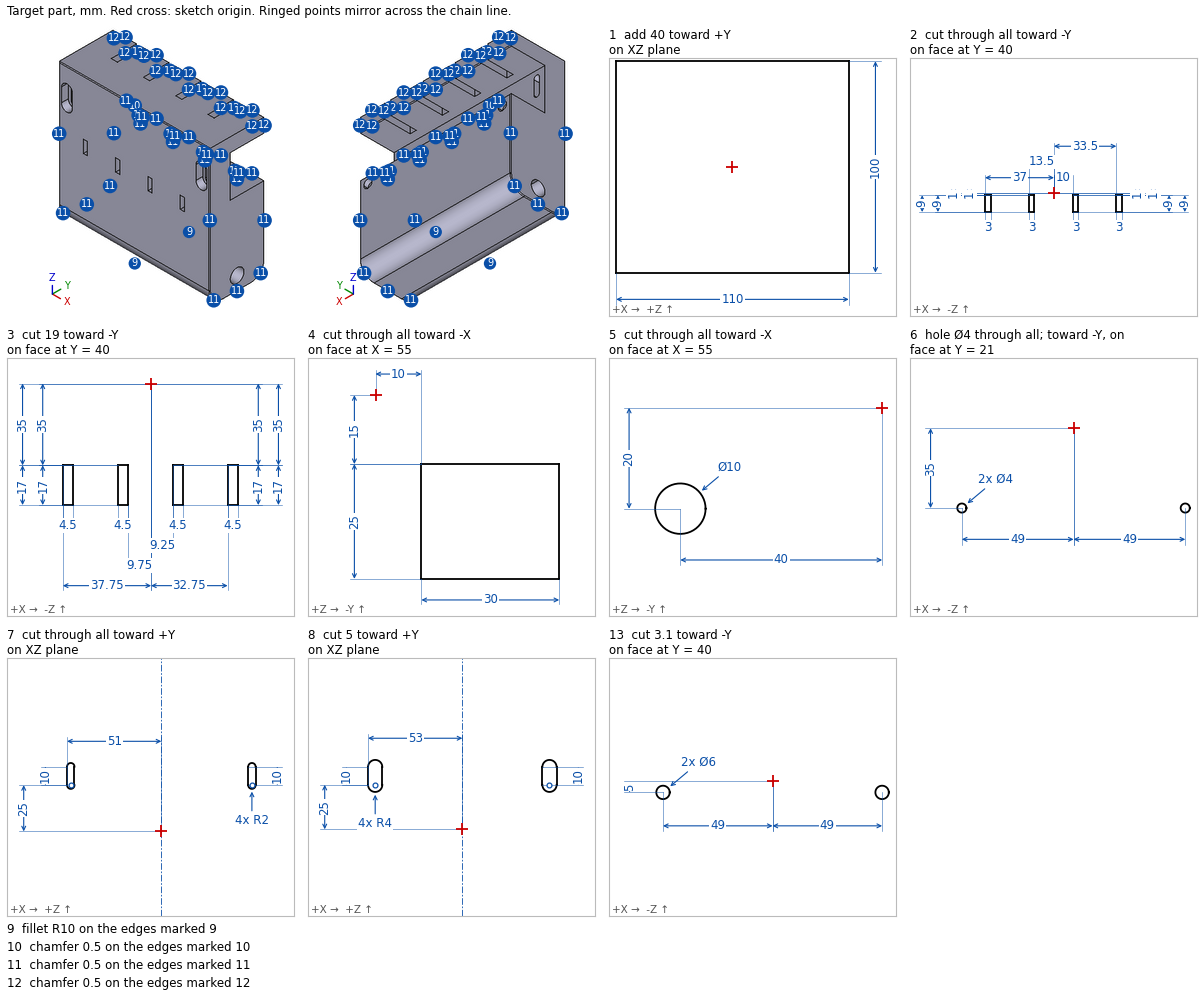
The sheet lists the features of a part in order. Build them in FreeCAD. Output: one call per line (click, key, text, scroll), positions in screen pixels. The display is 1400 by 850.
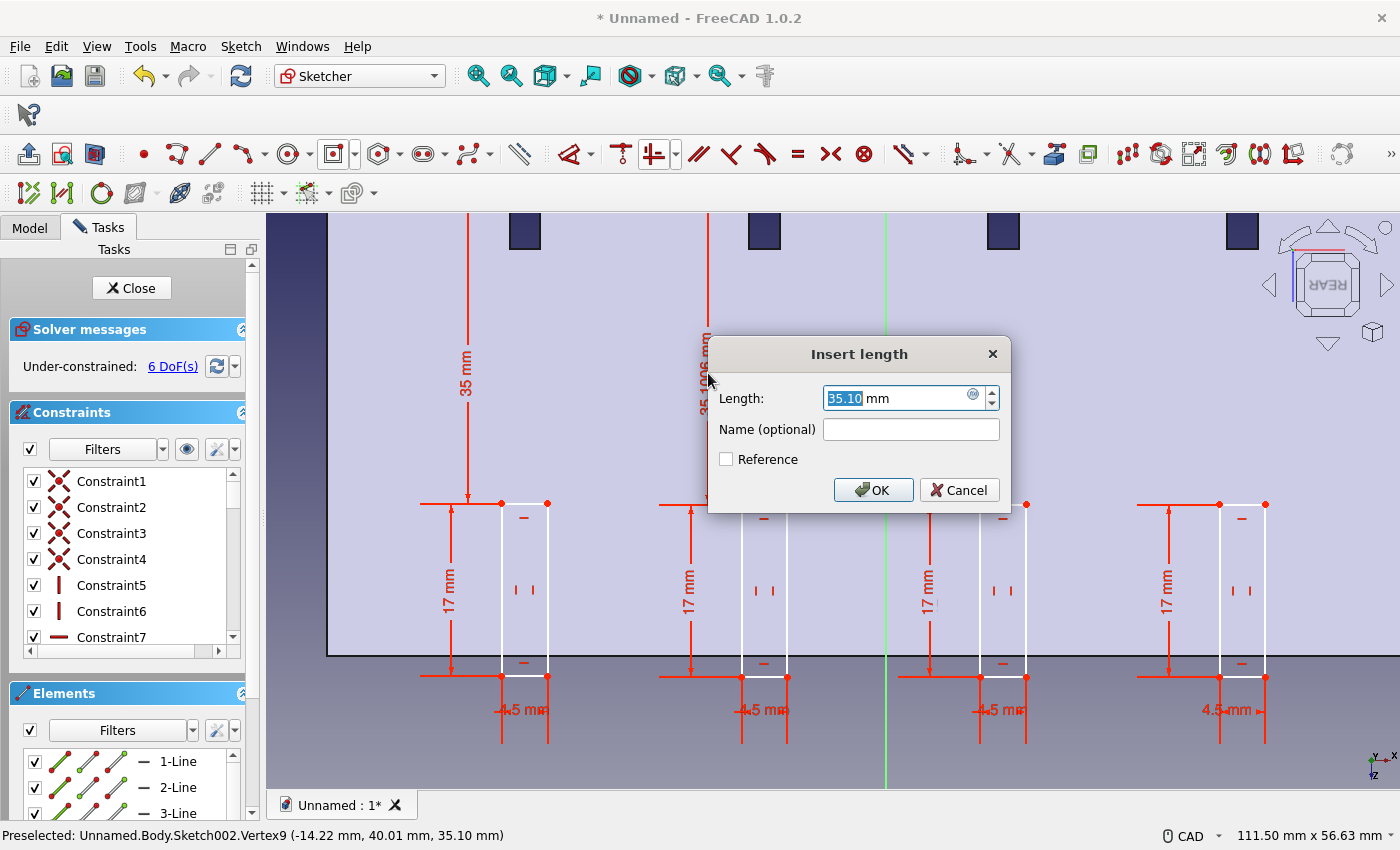
text(35)
key(Return)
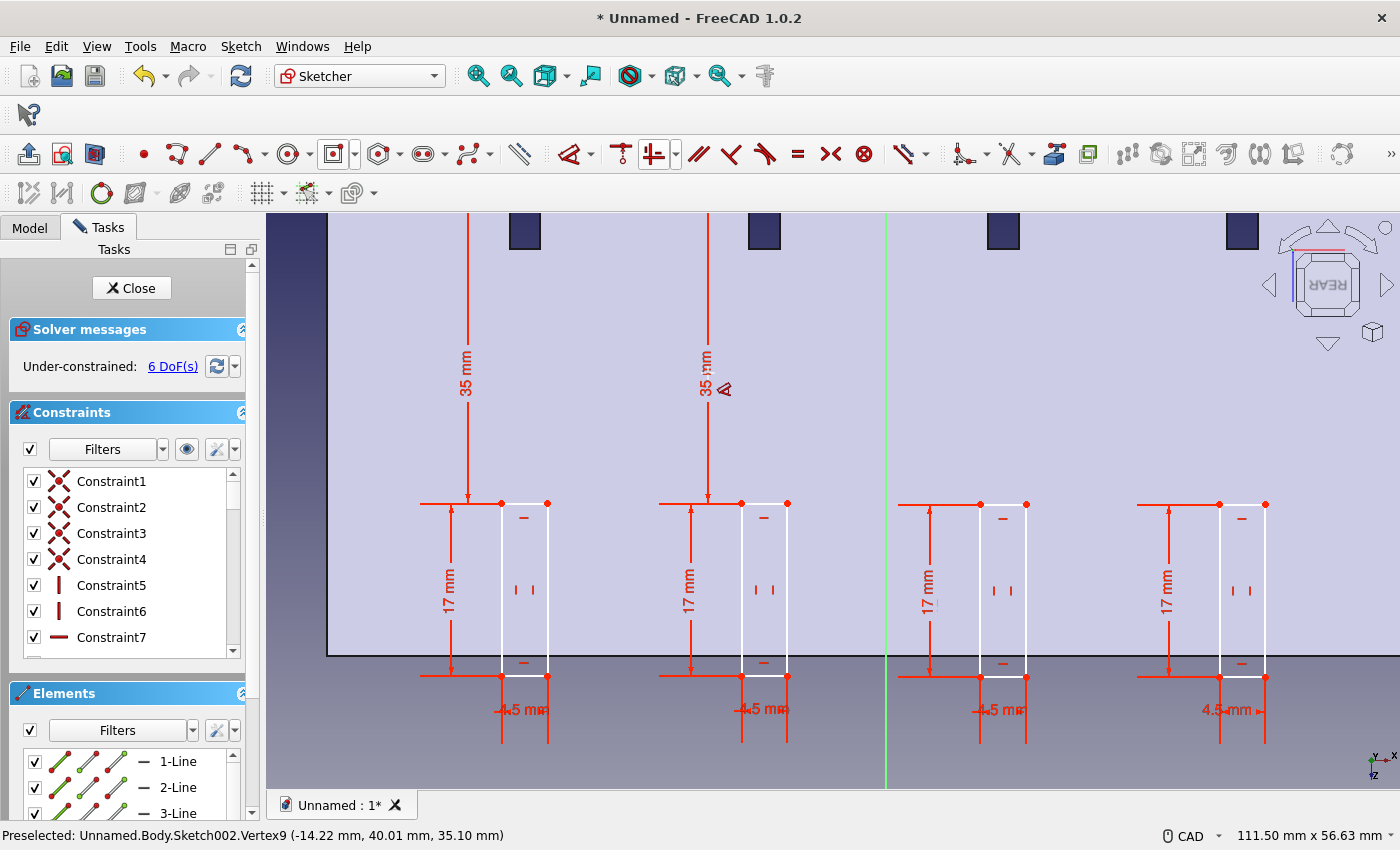
click(980, 505)
click(1014, 373)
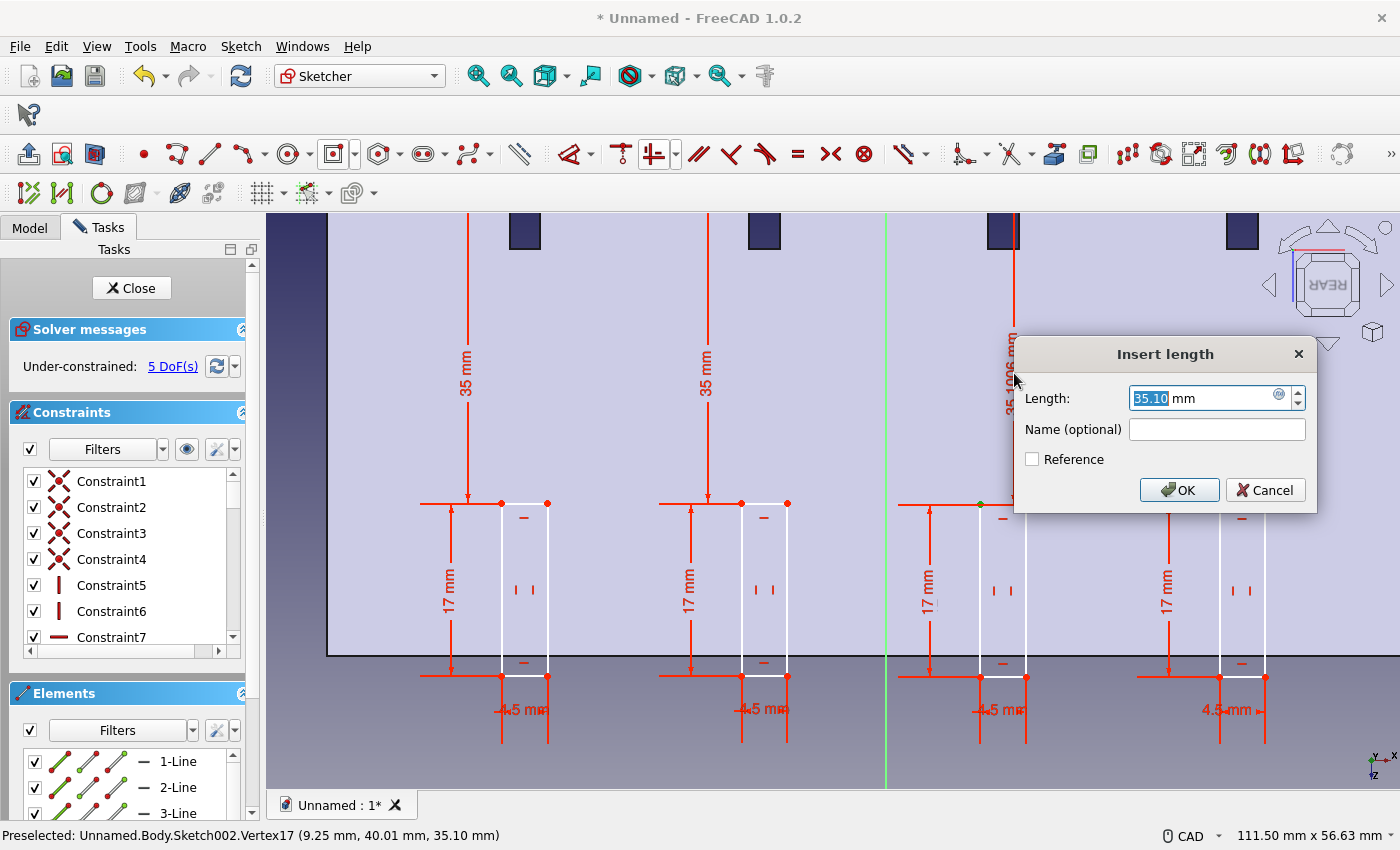
text(35)
key(Return)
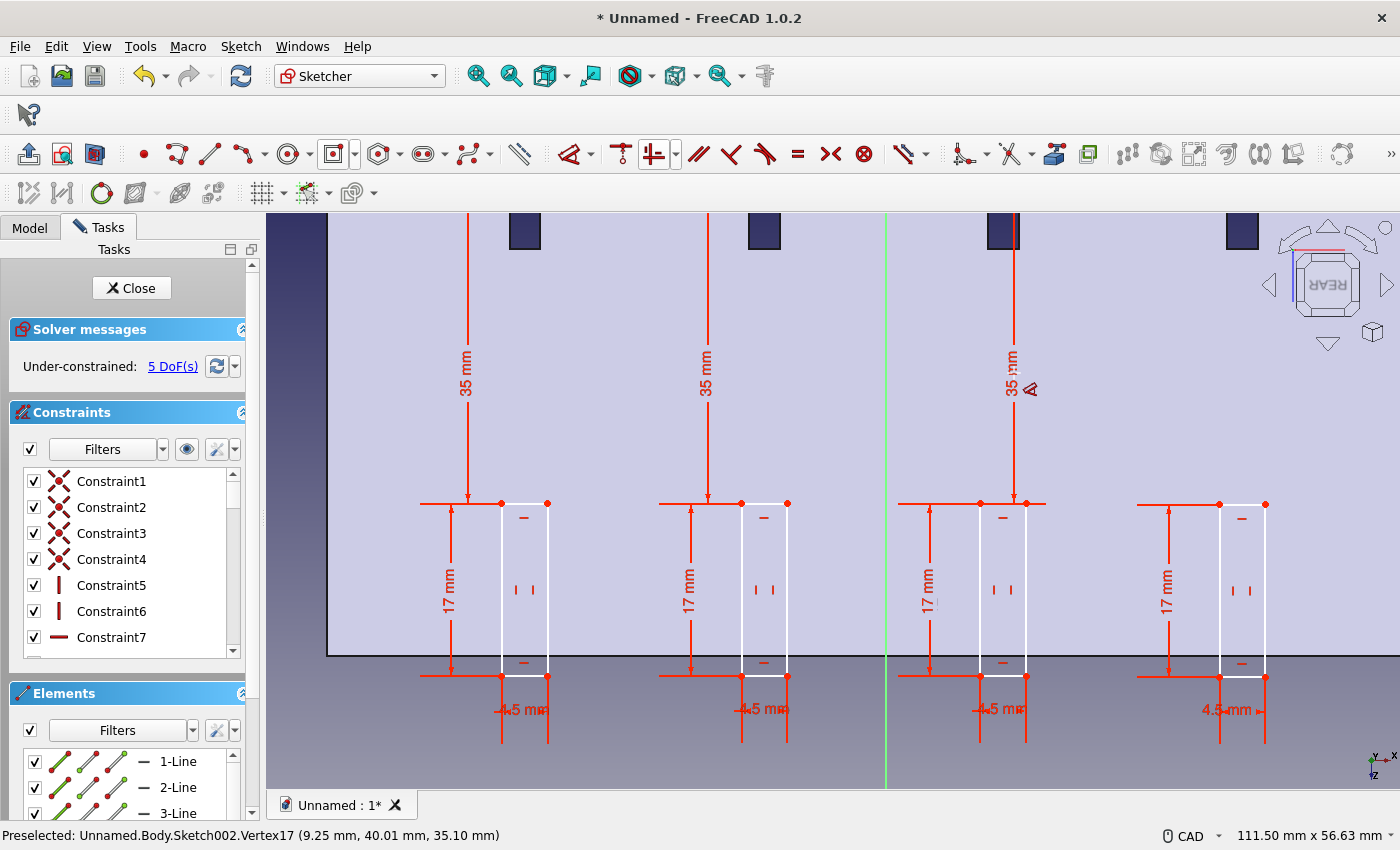
click(1220, 505)
click(852, 373)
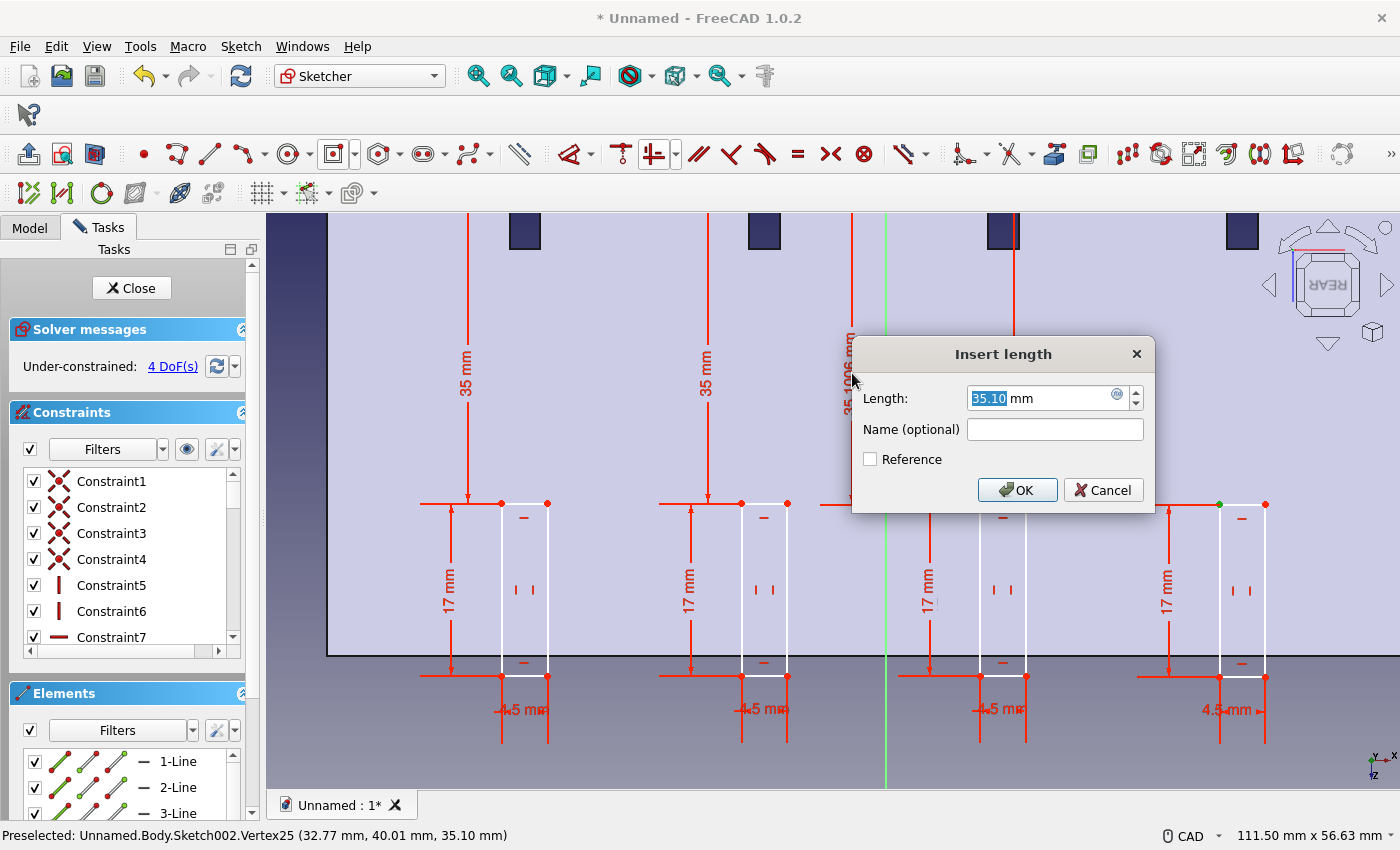
text(35)
key(Return)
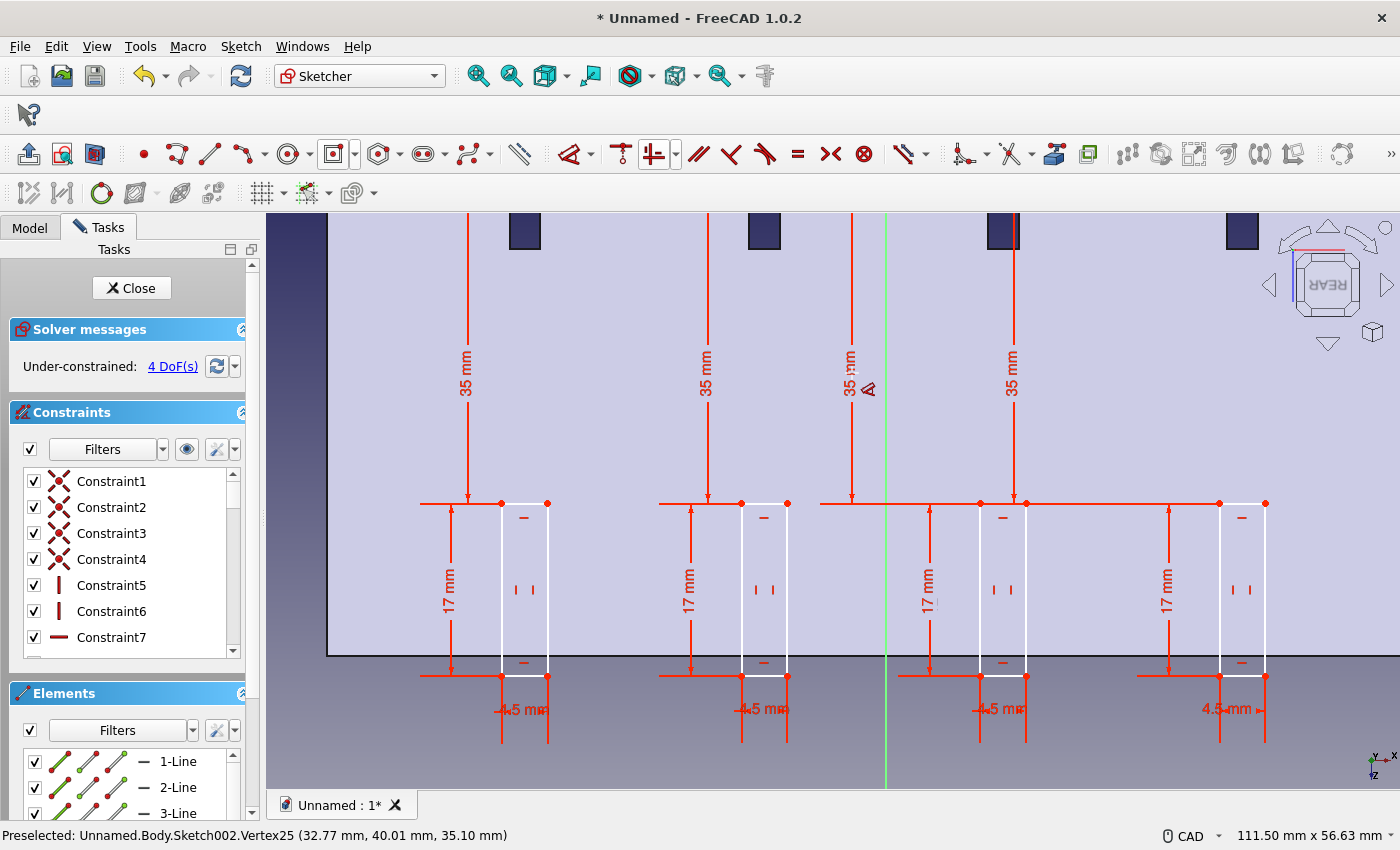
click(787, 676)
click(837, 710)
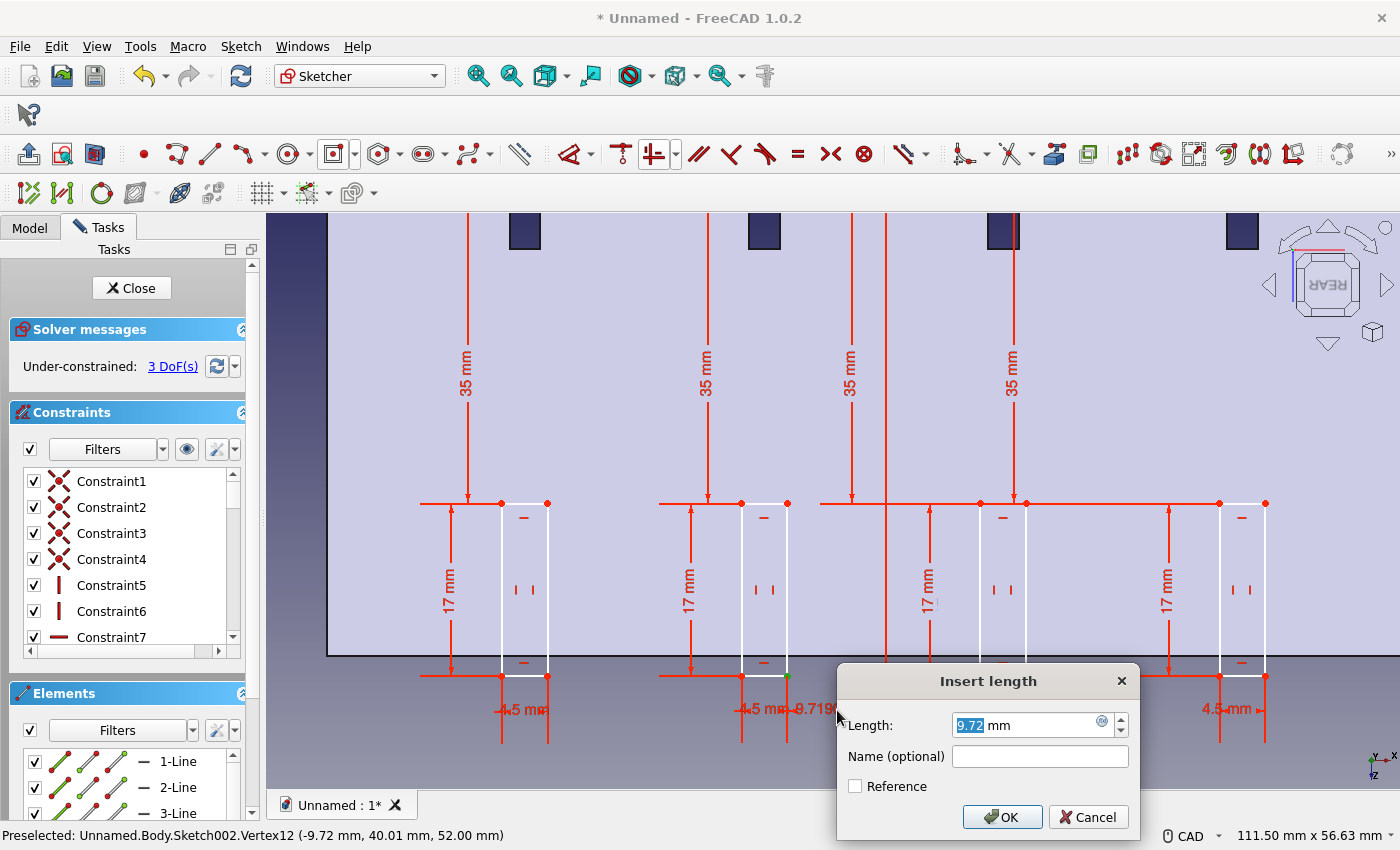
text(9.75)
key(Return)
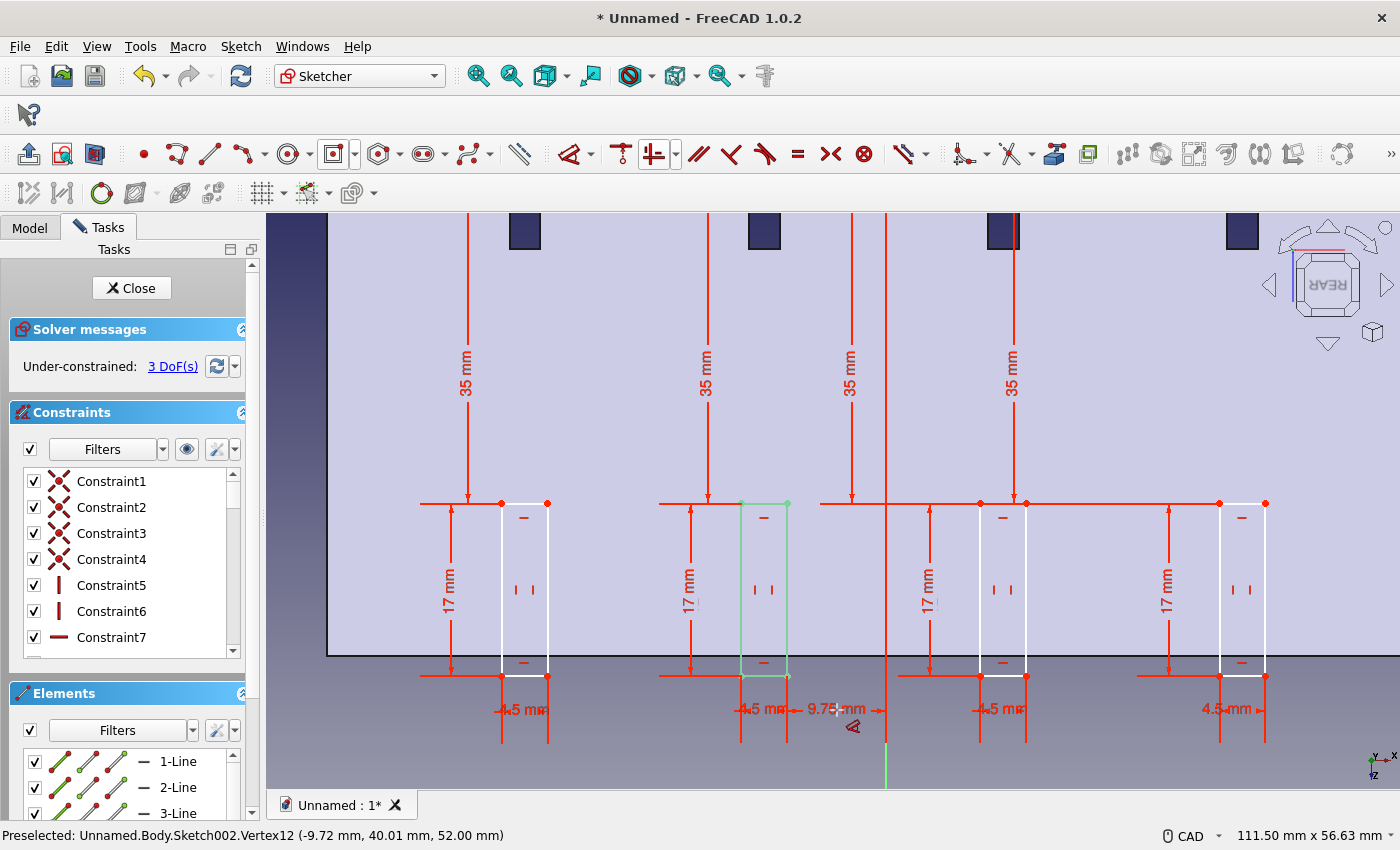
click(980, 504)
click(933, 538)